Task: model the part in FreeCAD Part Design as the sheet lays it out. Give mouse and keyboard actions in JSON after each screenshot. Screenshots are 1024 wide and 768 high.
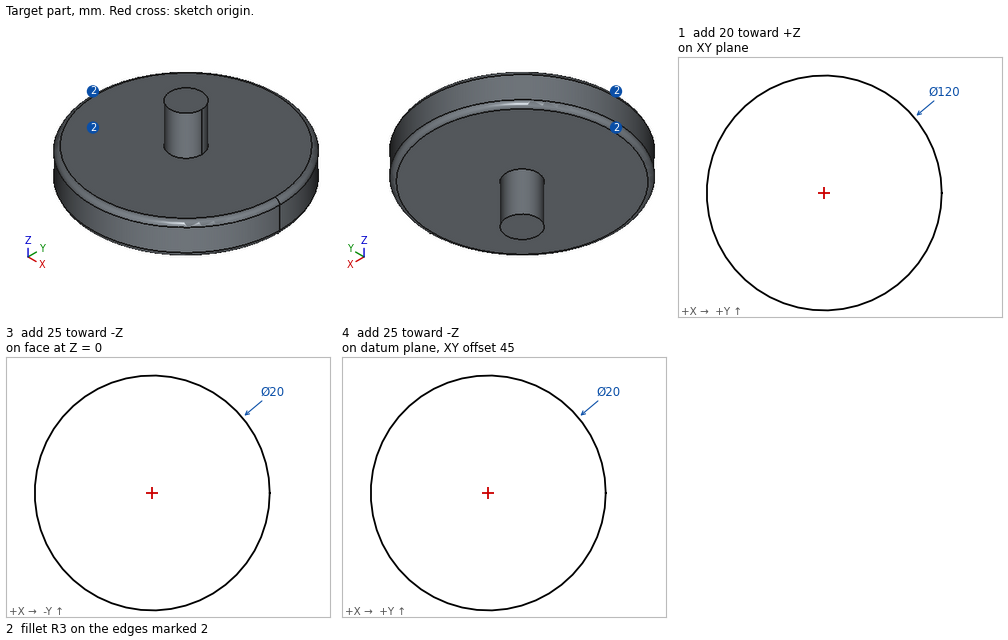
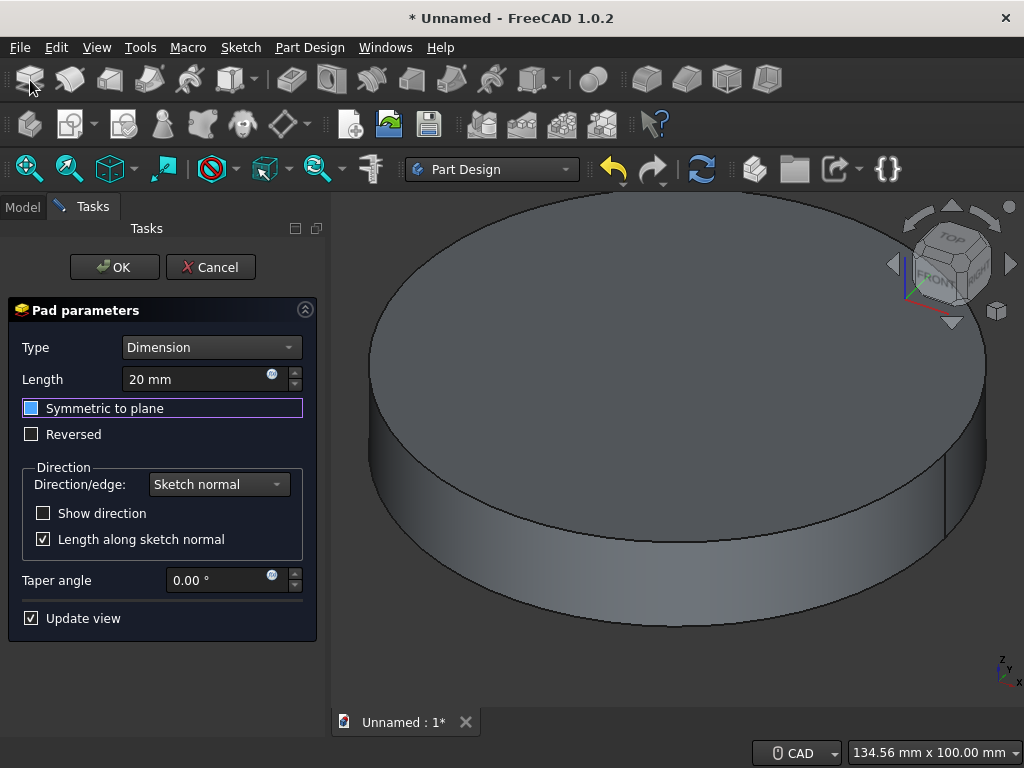
{"action": "left_click", "coordinate": [115, 267]}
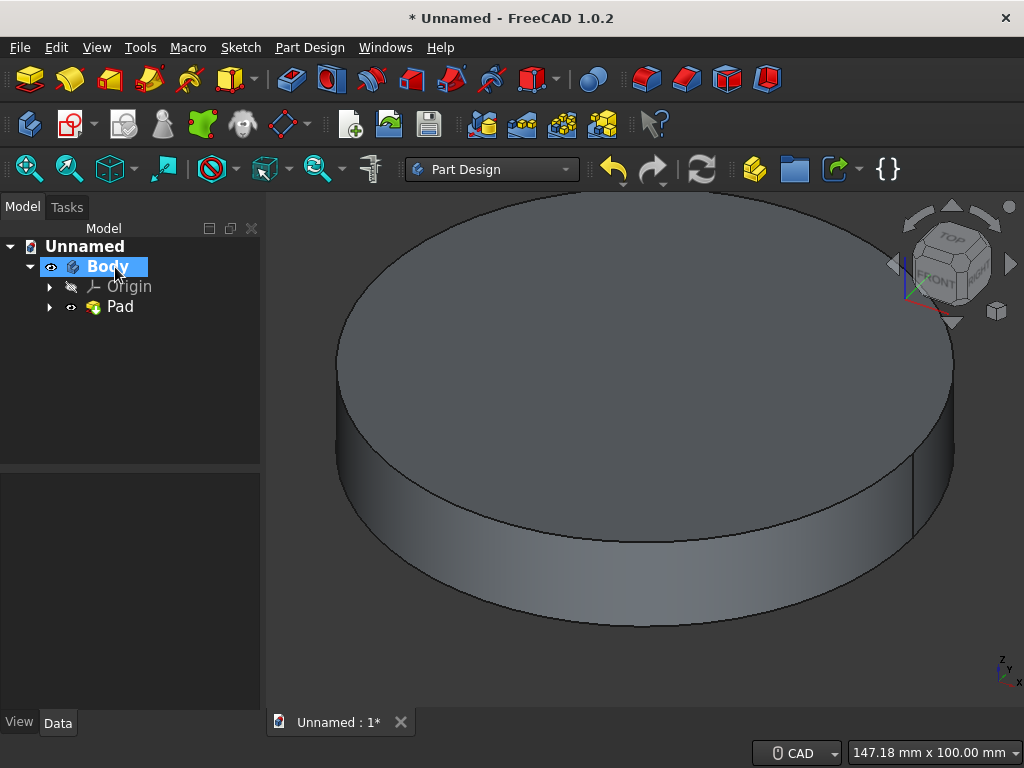
{"action": "key", "text": "v f"}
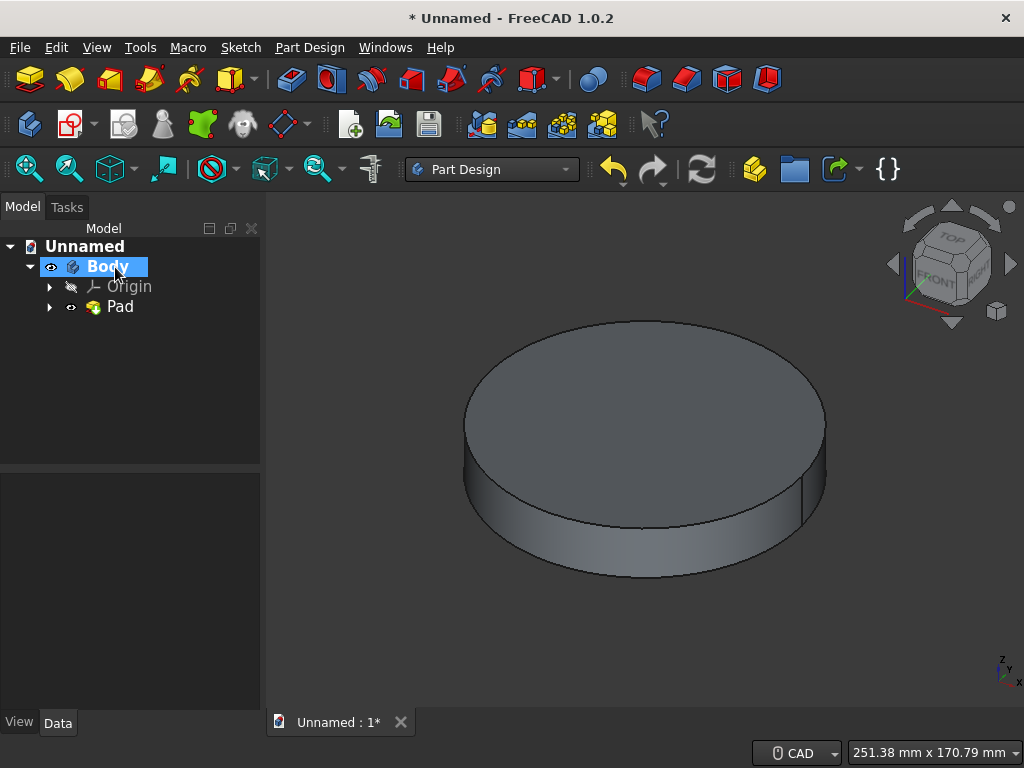
{"action": "left_click", "coordinate": [465, 435]}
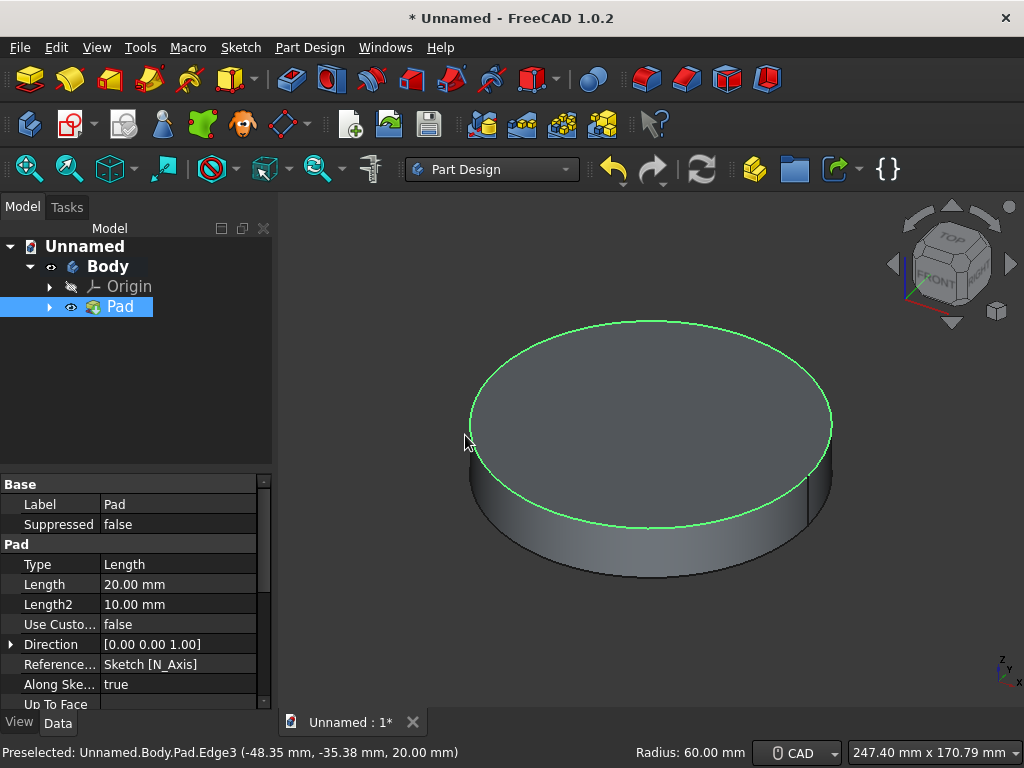
{"action": "key", "text": "0"}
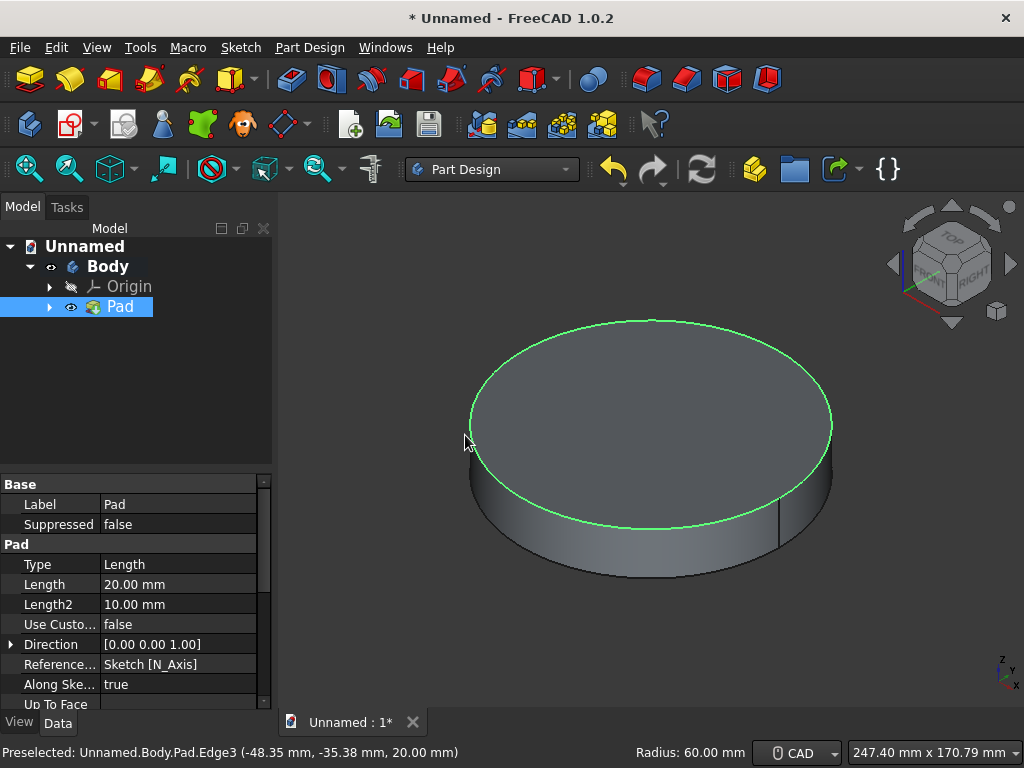
{"action": "key", "text": "2"}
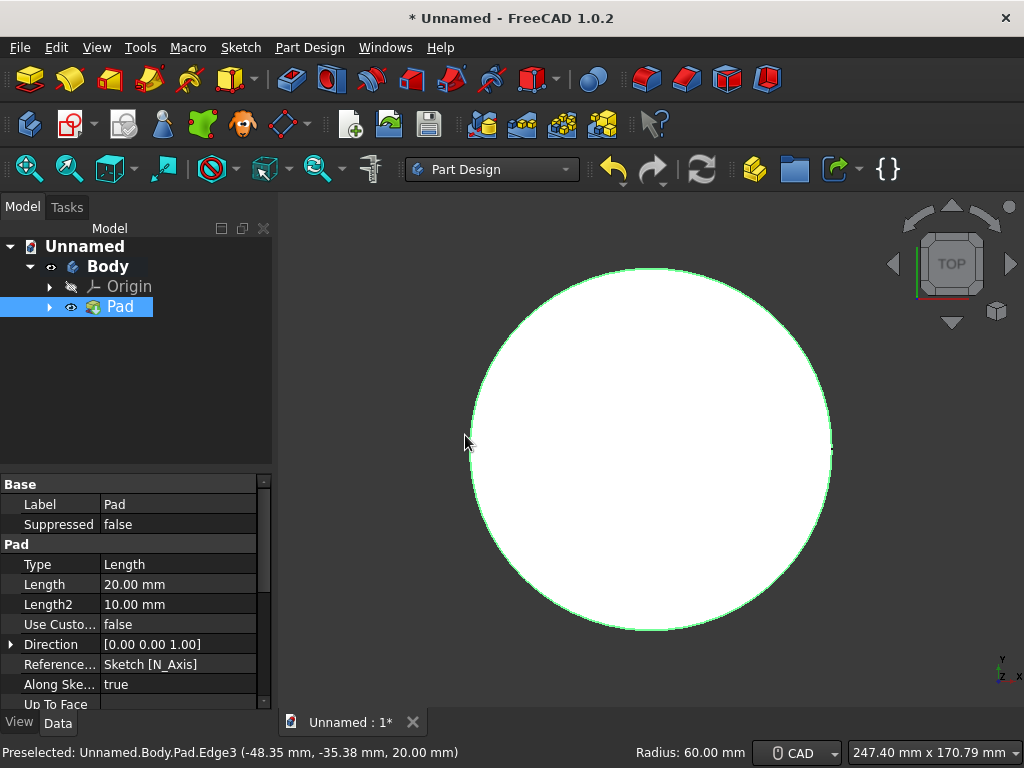
{"action": "key", "text": "1"}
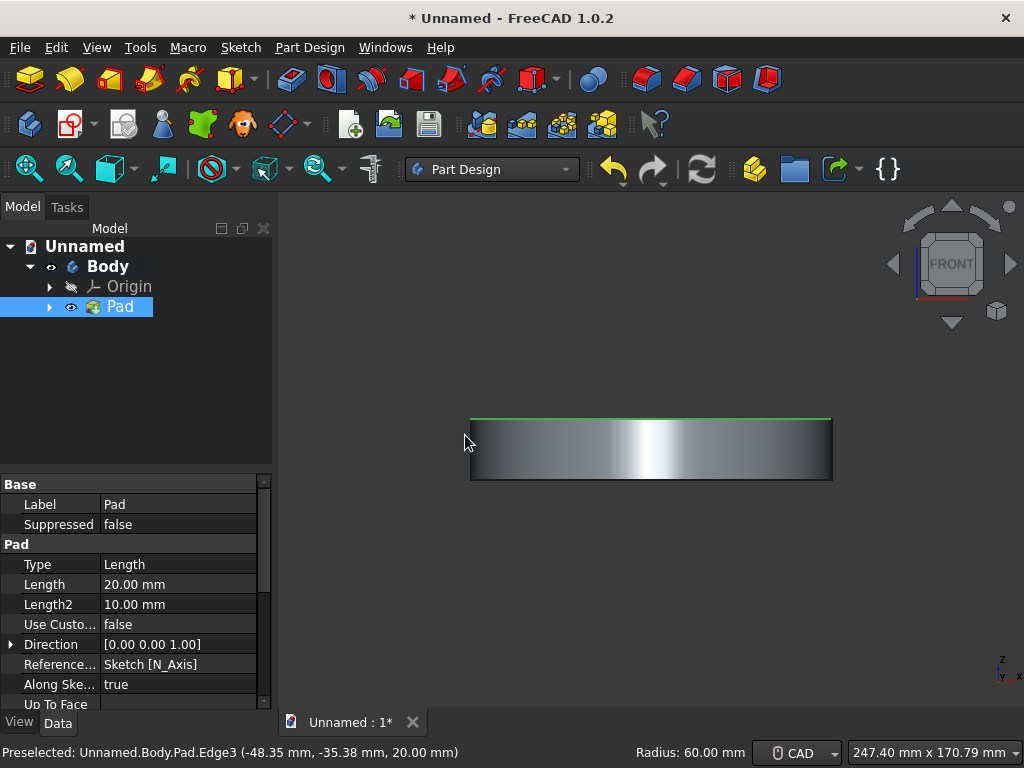
{"action": "left_click", "coordinate": [505, 479], "text": "ctrl"}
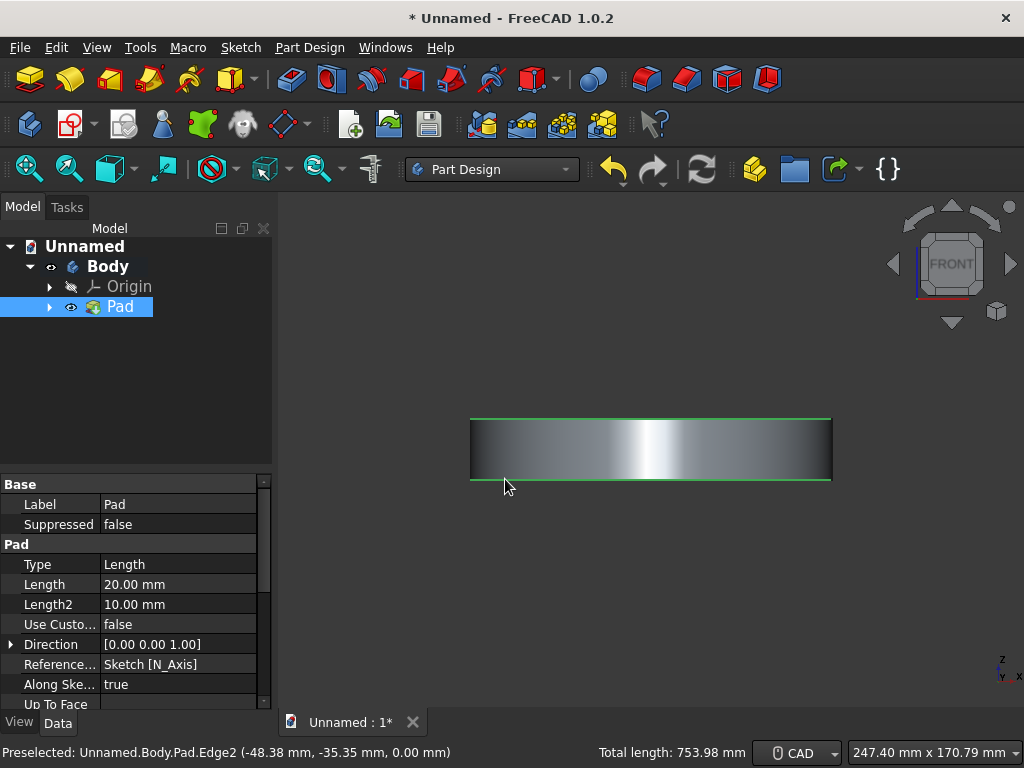
{"action": "left_click", "coordinate": [648, 80]}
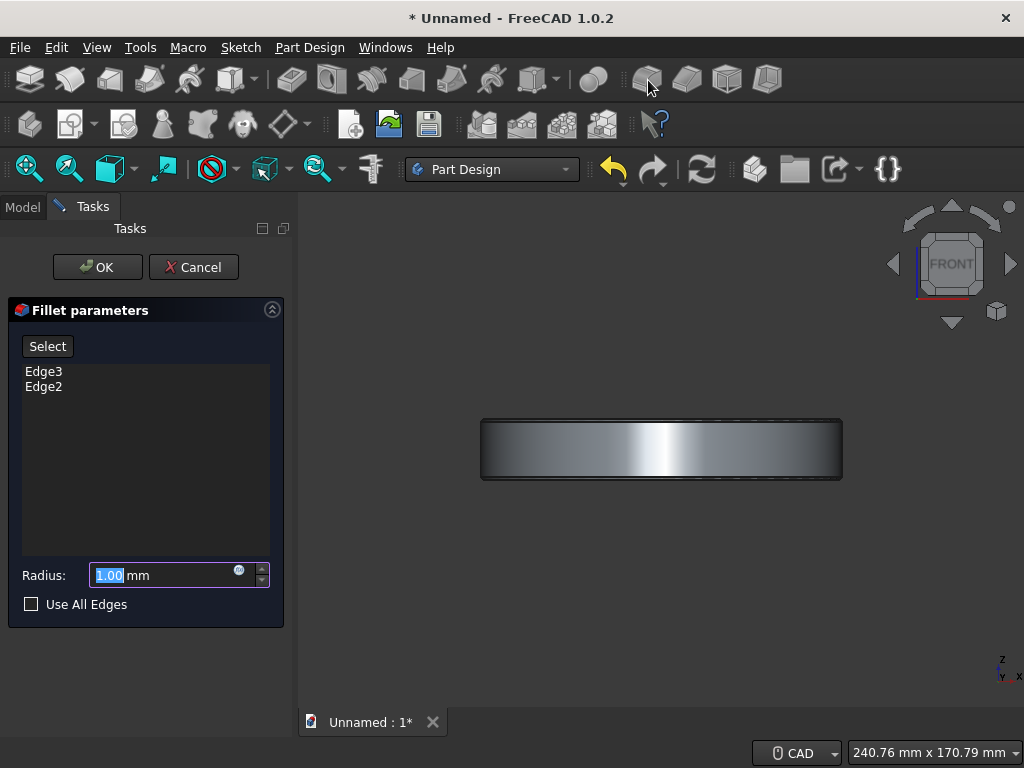
{"action": "type", "text": "3"}
{"action": "key", "text": "Tab"}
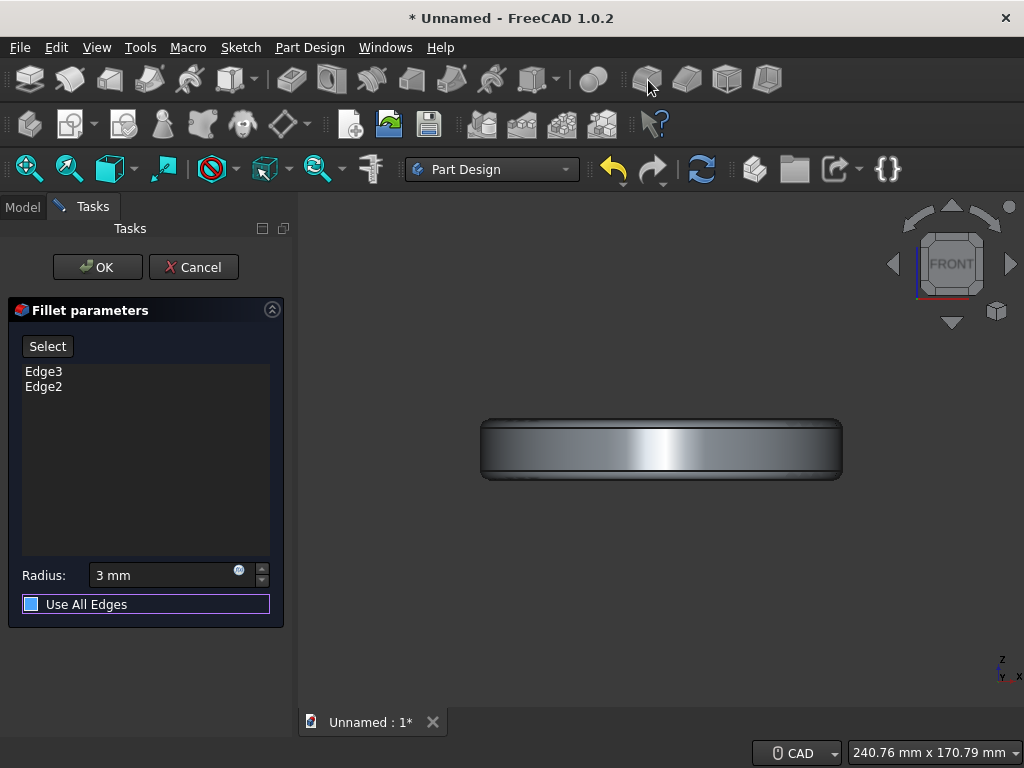
{"action": "left_click", "coordinate": [98, 267]}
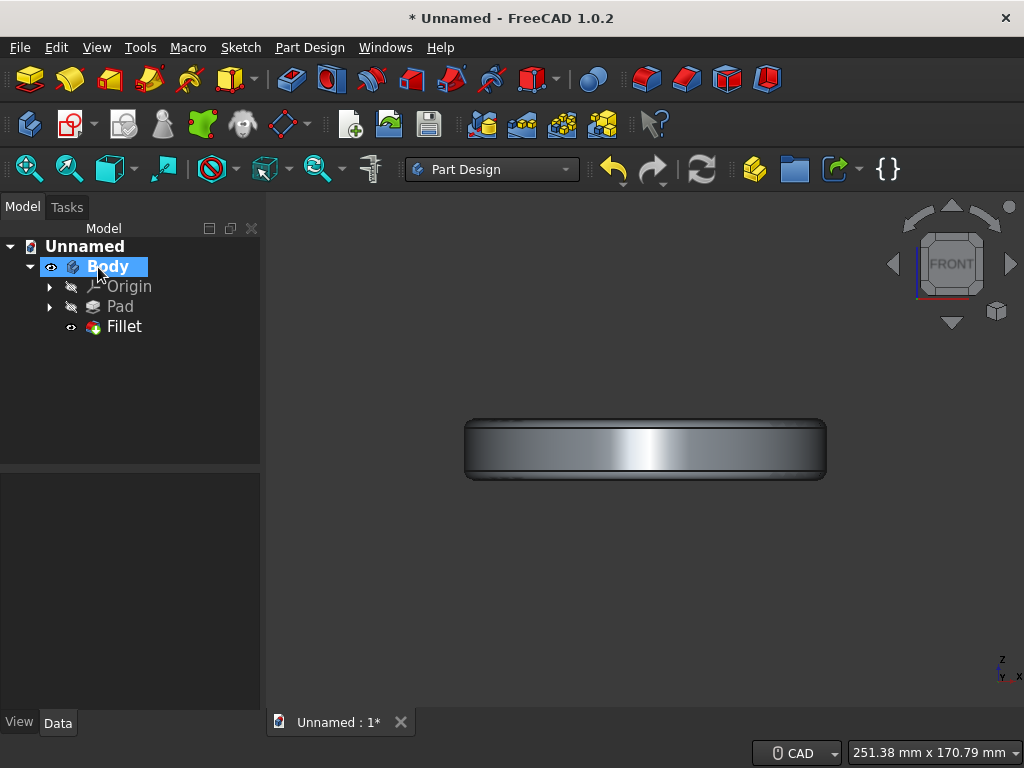
{"action": "key", "text": "5"}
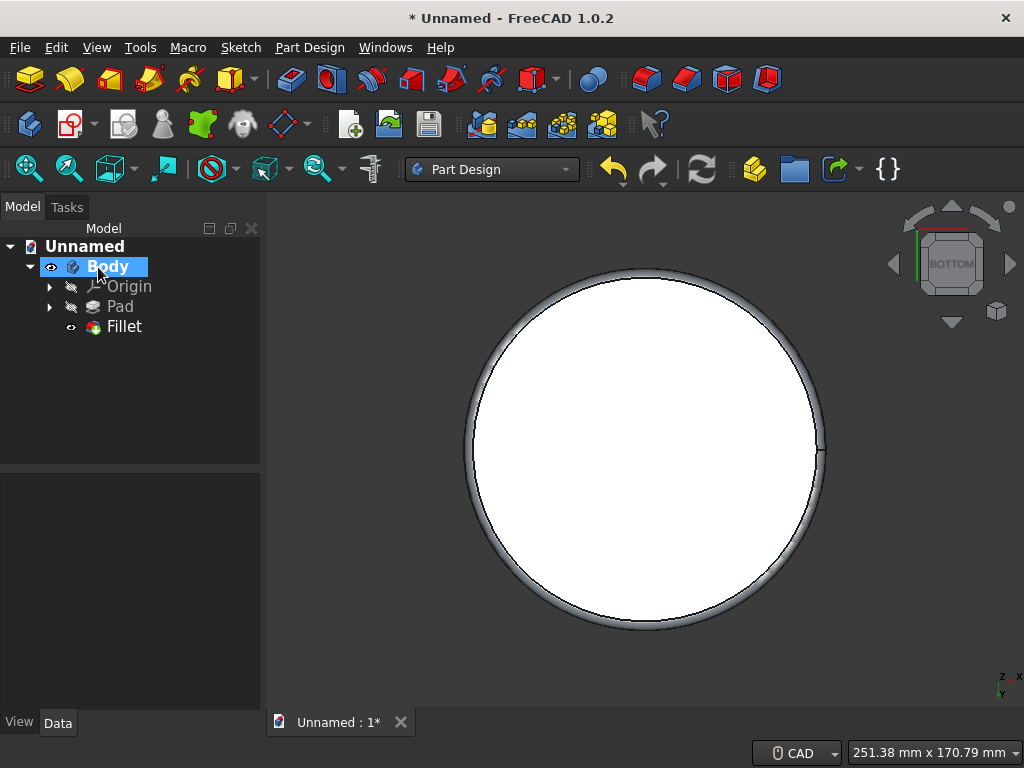
{"action": "left_click", "coordinate": [645, 448]}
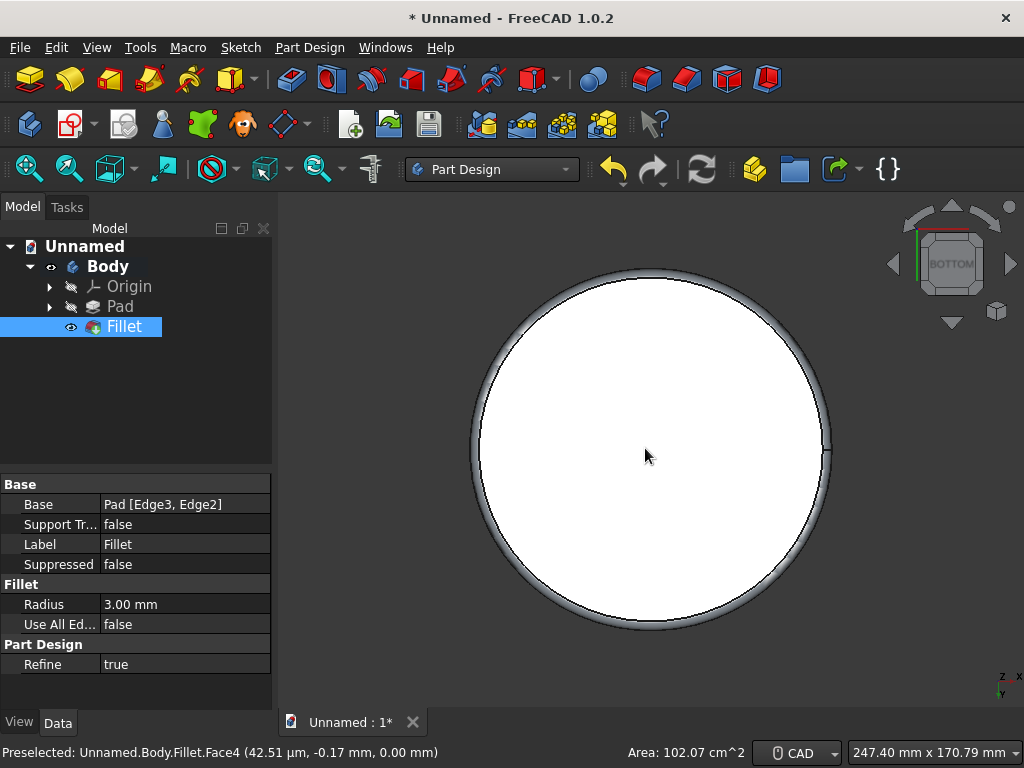
{"action": "left_click", "coordinate": [70, 124]}